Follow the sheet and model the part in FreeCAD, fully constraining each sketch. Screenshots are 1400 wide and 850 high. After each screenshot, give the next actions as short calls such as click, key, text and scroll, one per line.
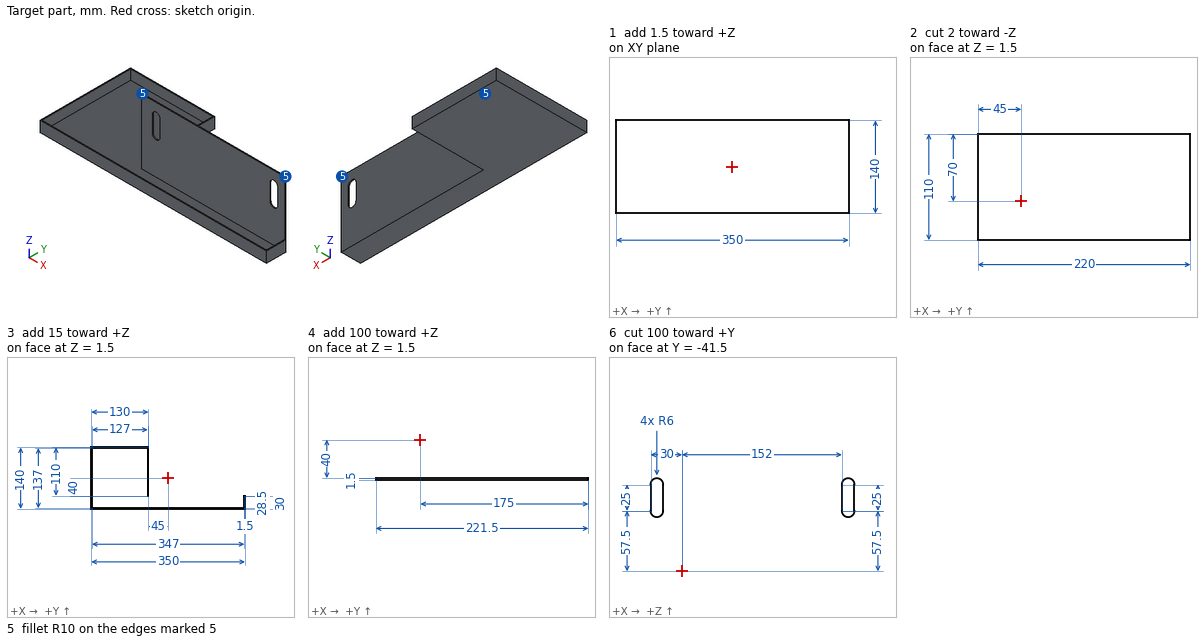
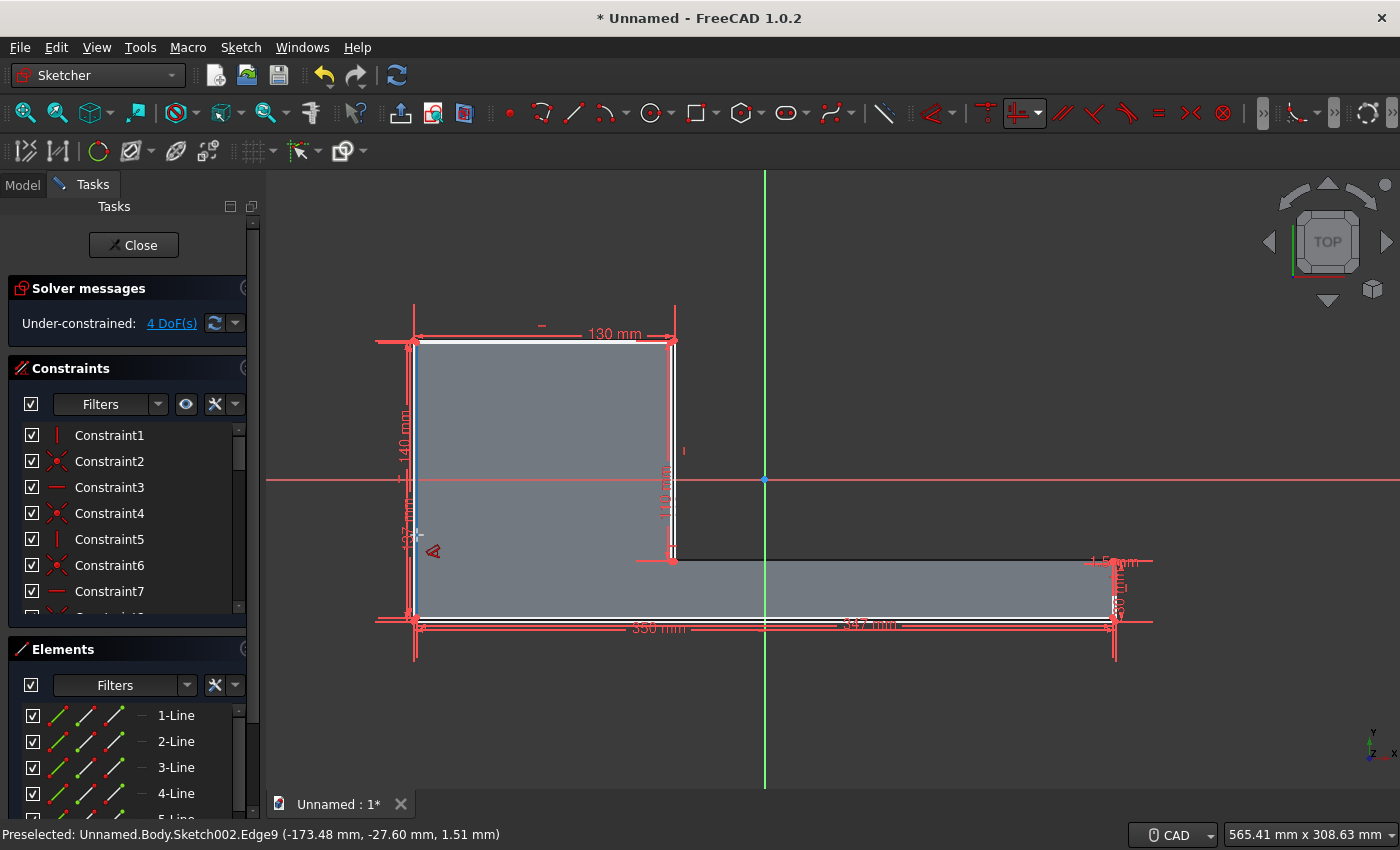
scroll(493, 343, up, 10)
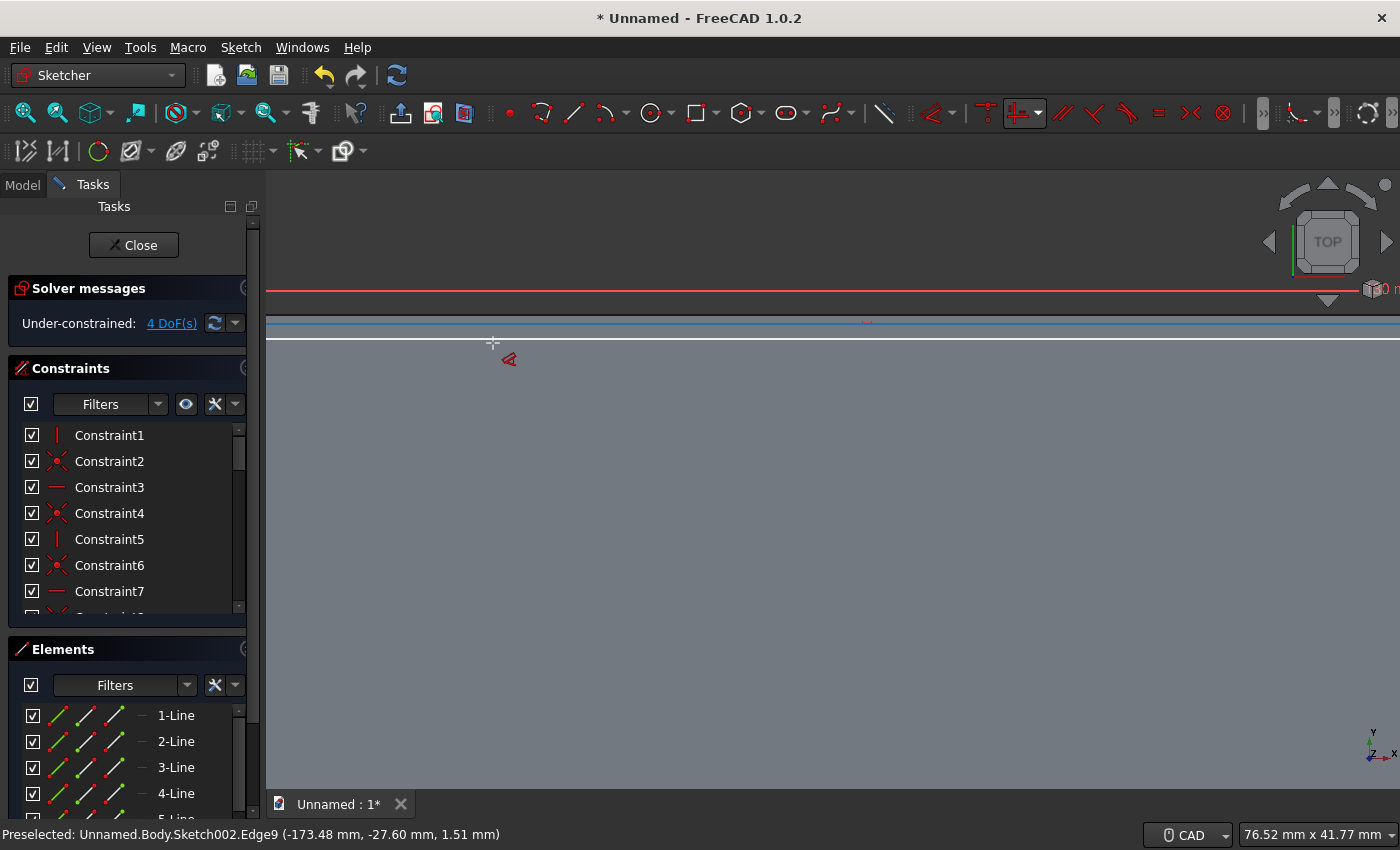
click(493, 339)
click(764, 305)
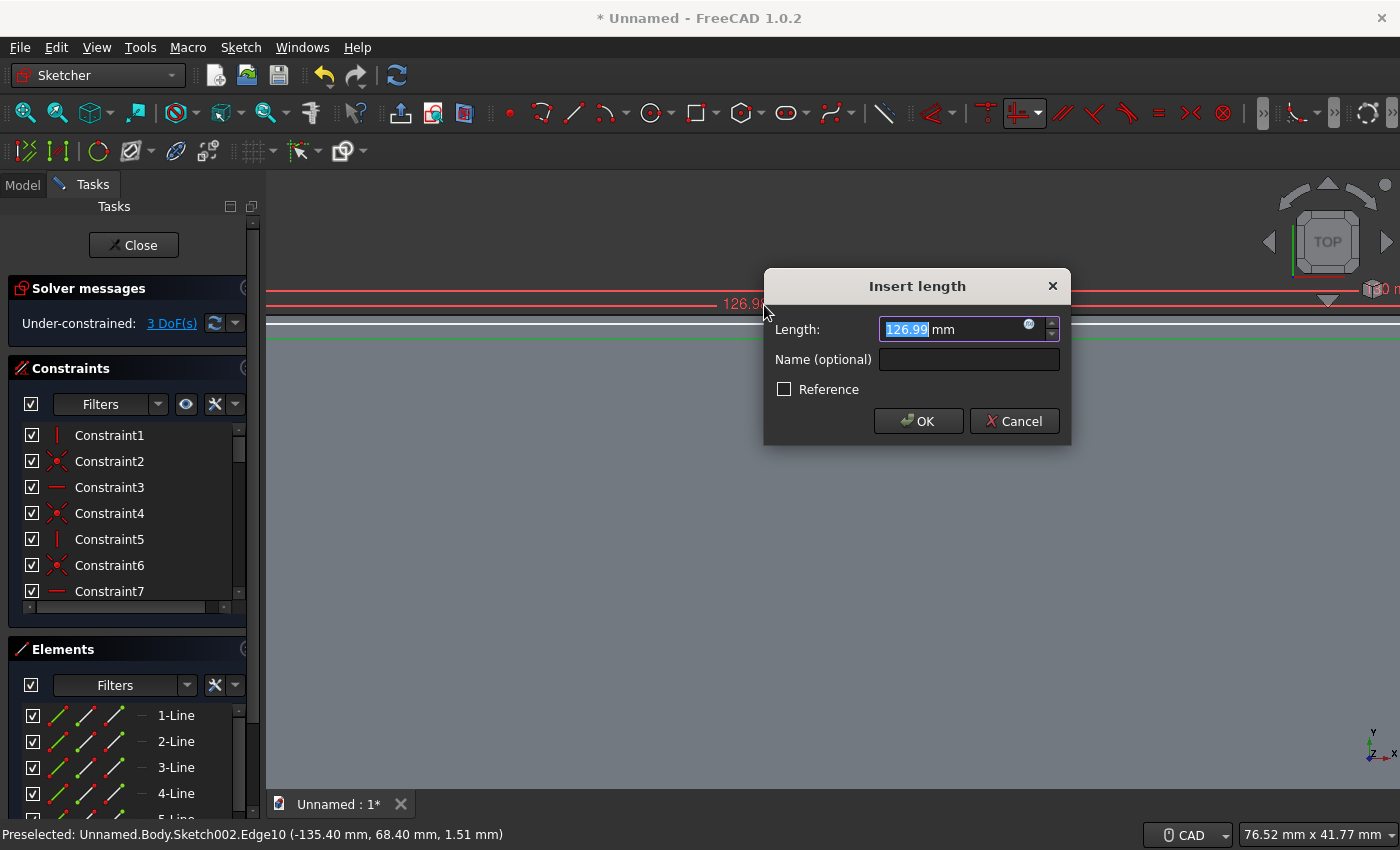
text(127)
key(Return)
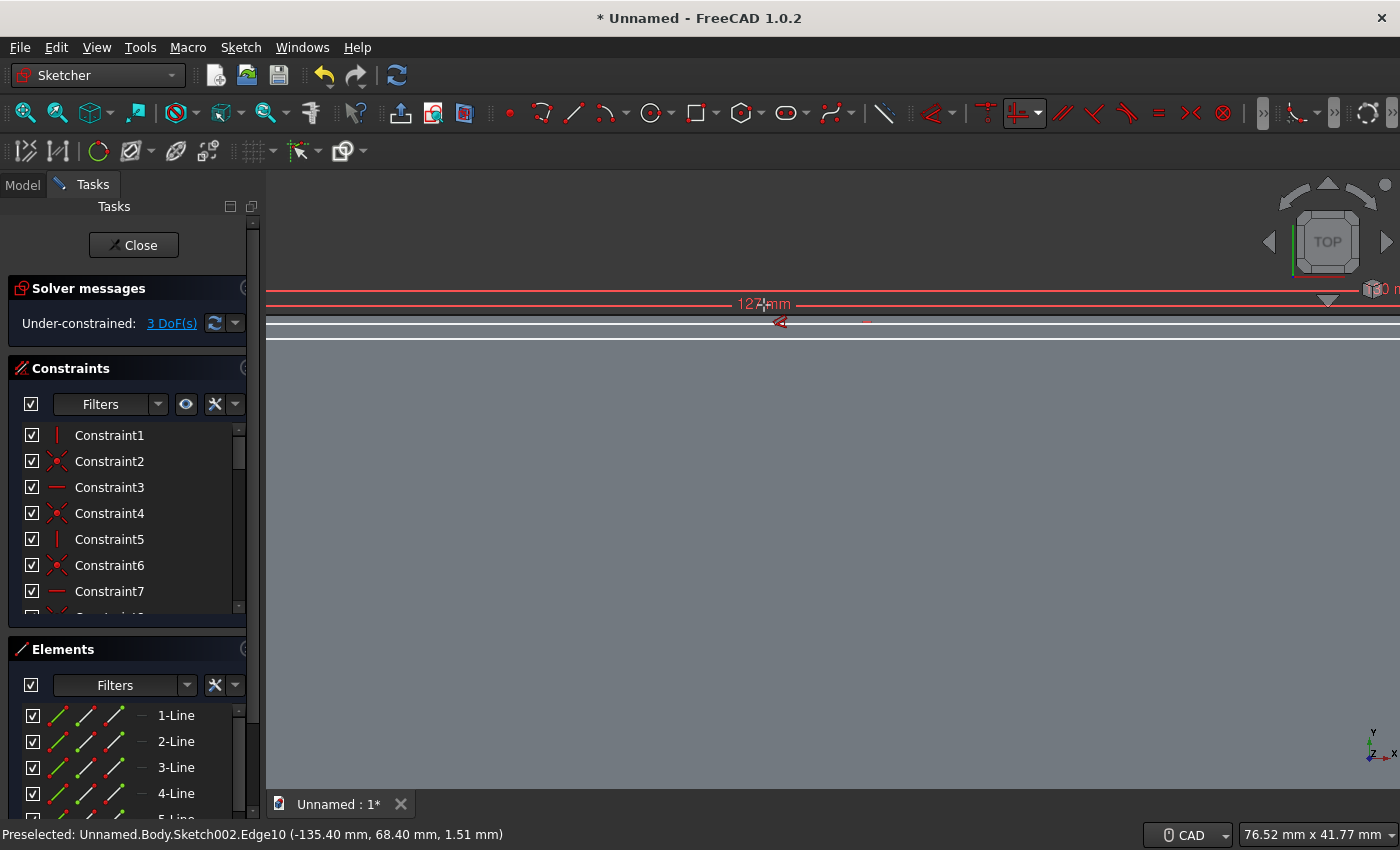
scroll(493, 343, down, 10)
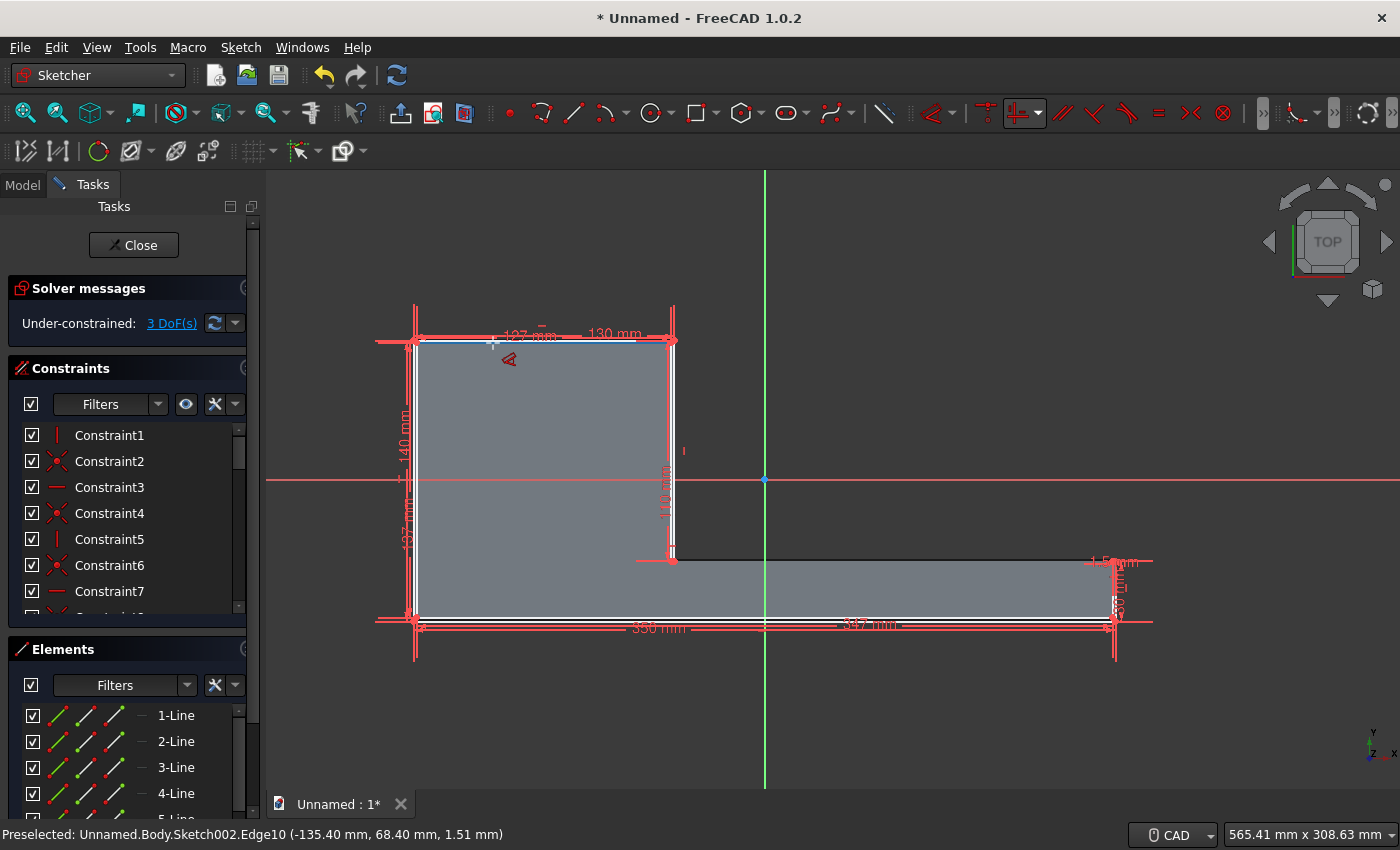
scroll(674, 561, up, 8)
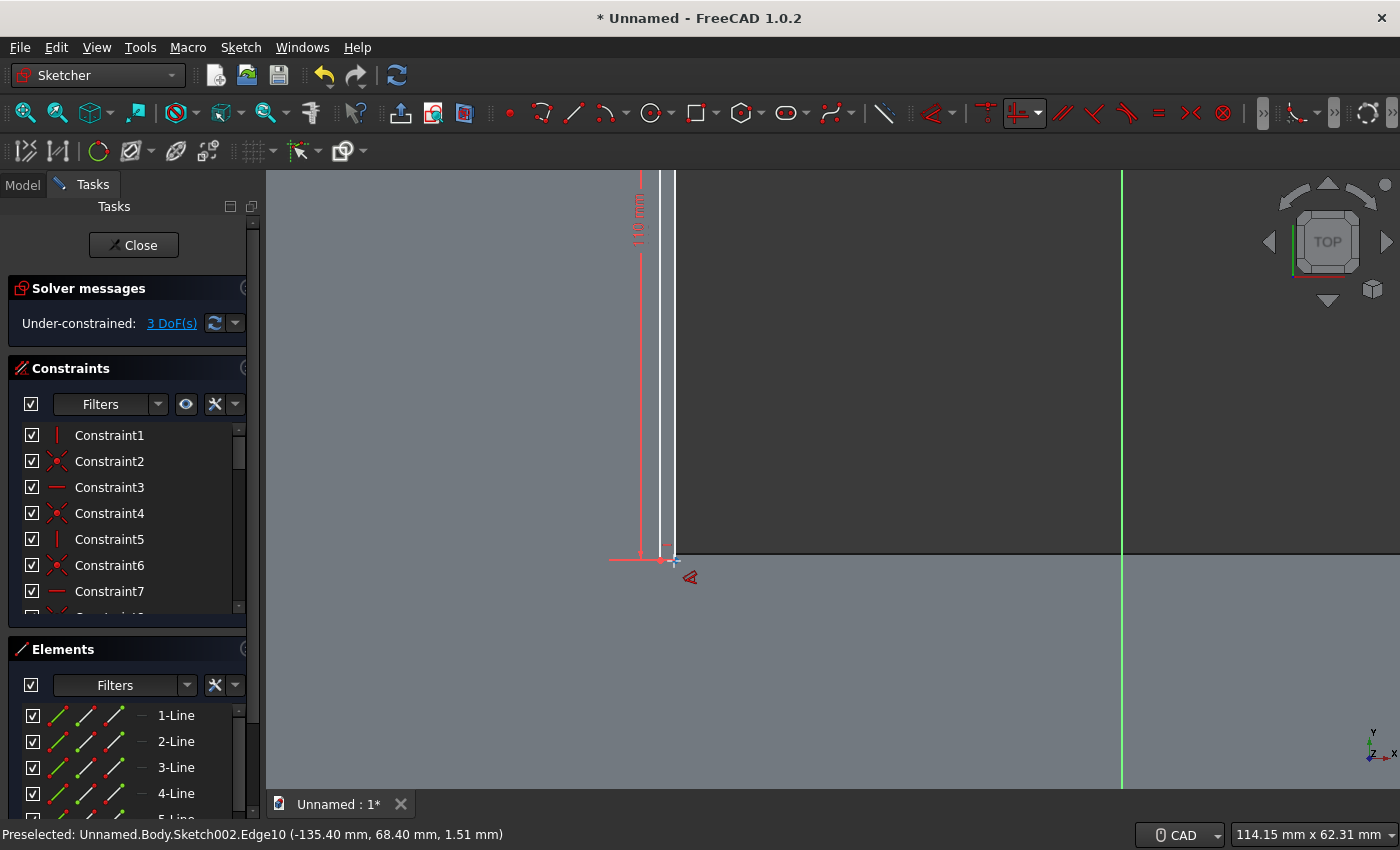
click(675, 560)
click(899, 594)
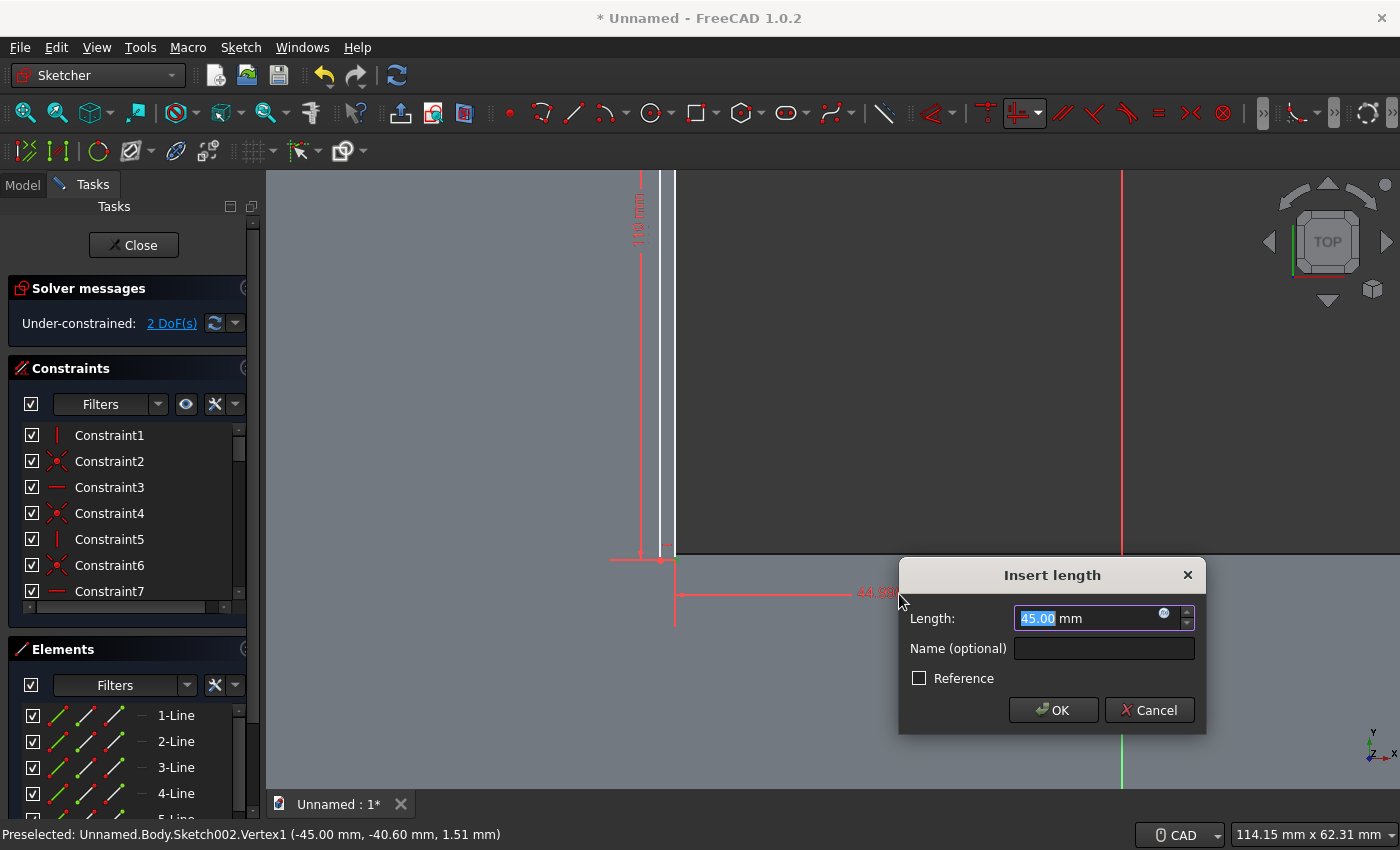
text(45)
key(Return)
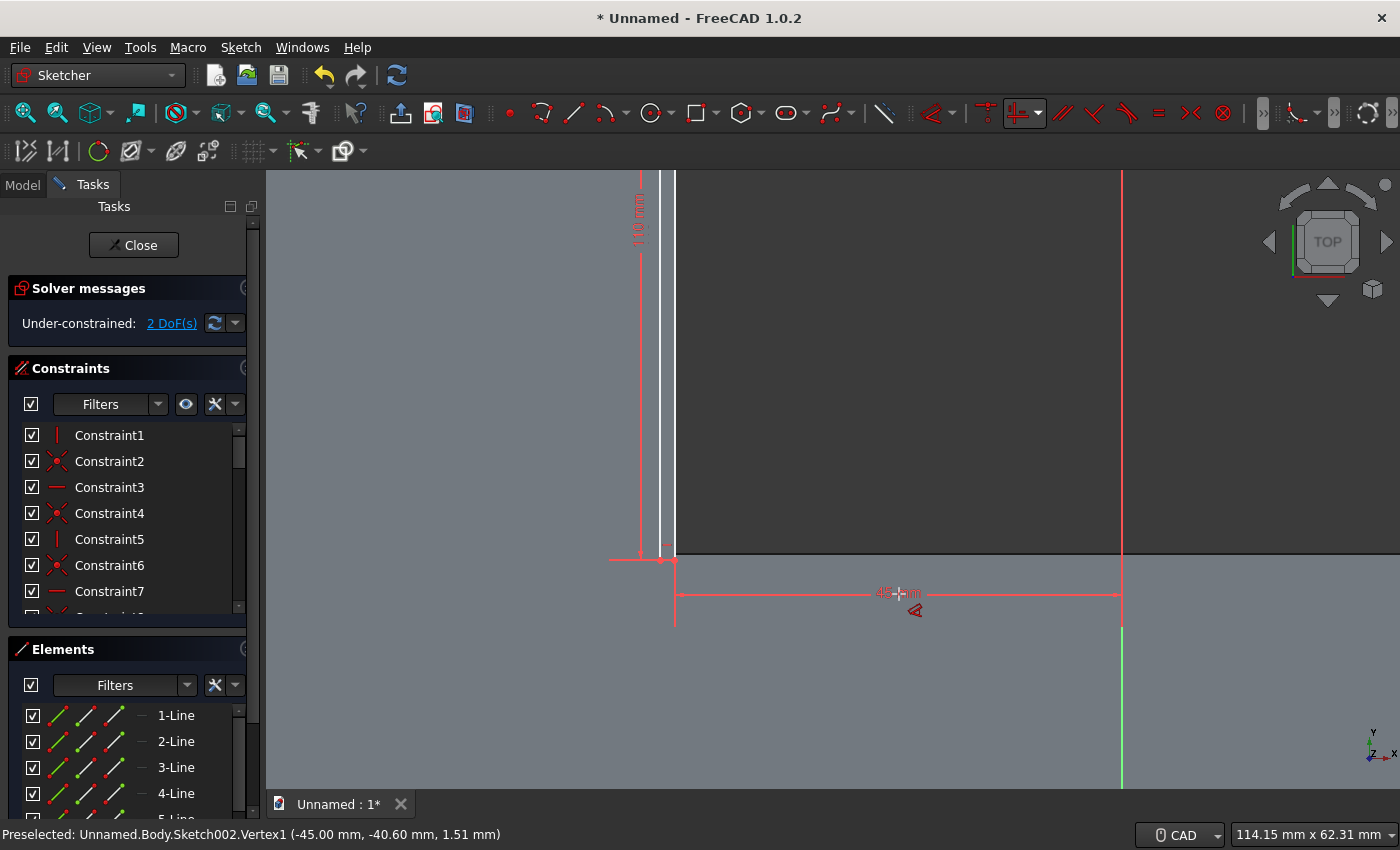
click(675, 560)
click(641, 379)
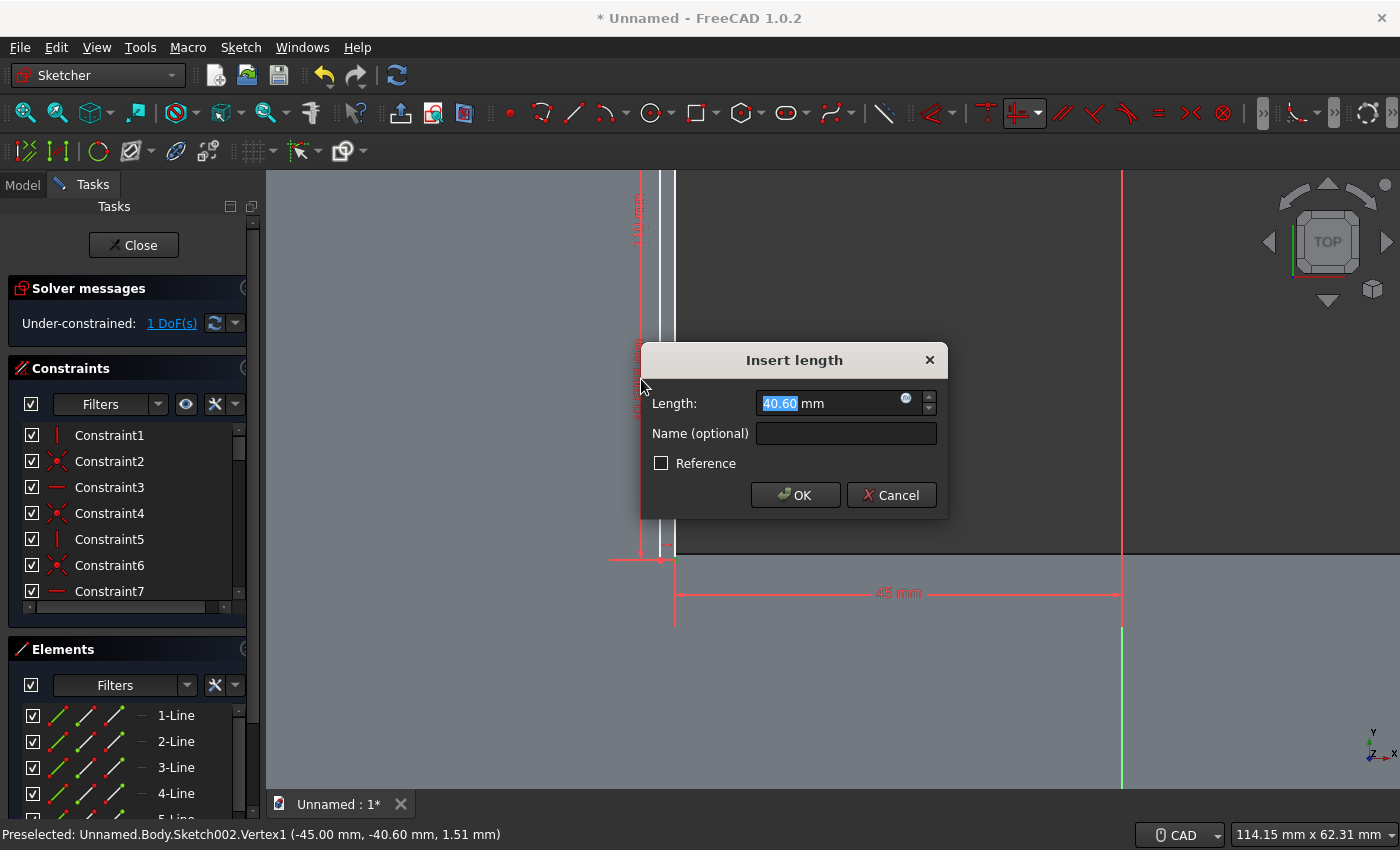
text(40)
key(Return)